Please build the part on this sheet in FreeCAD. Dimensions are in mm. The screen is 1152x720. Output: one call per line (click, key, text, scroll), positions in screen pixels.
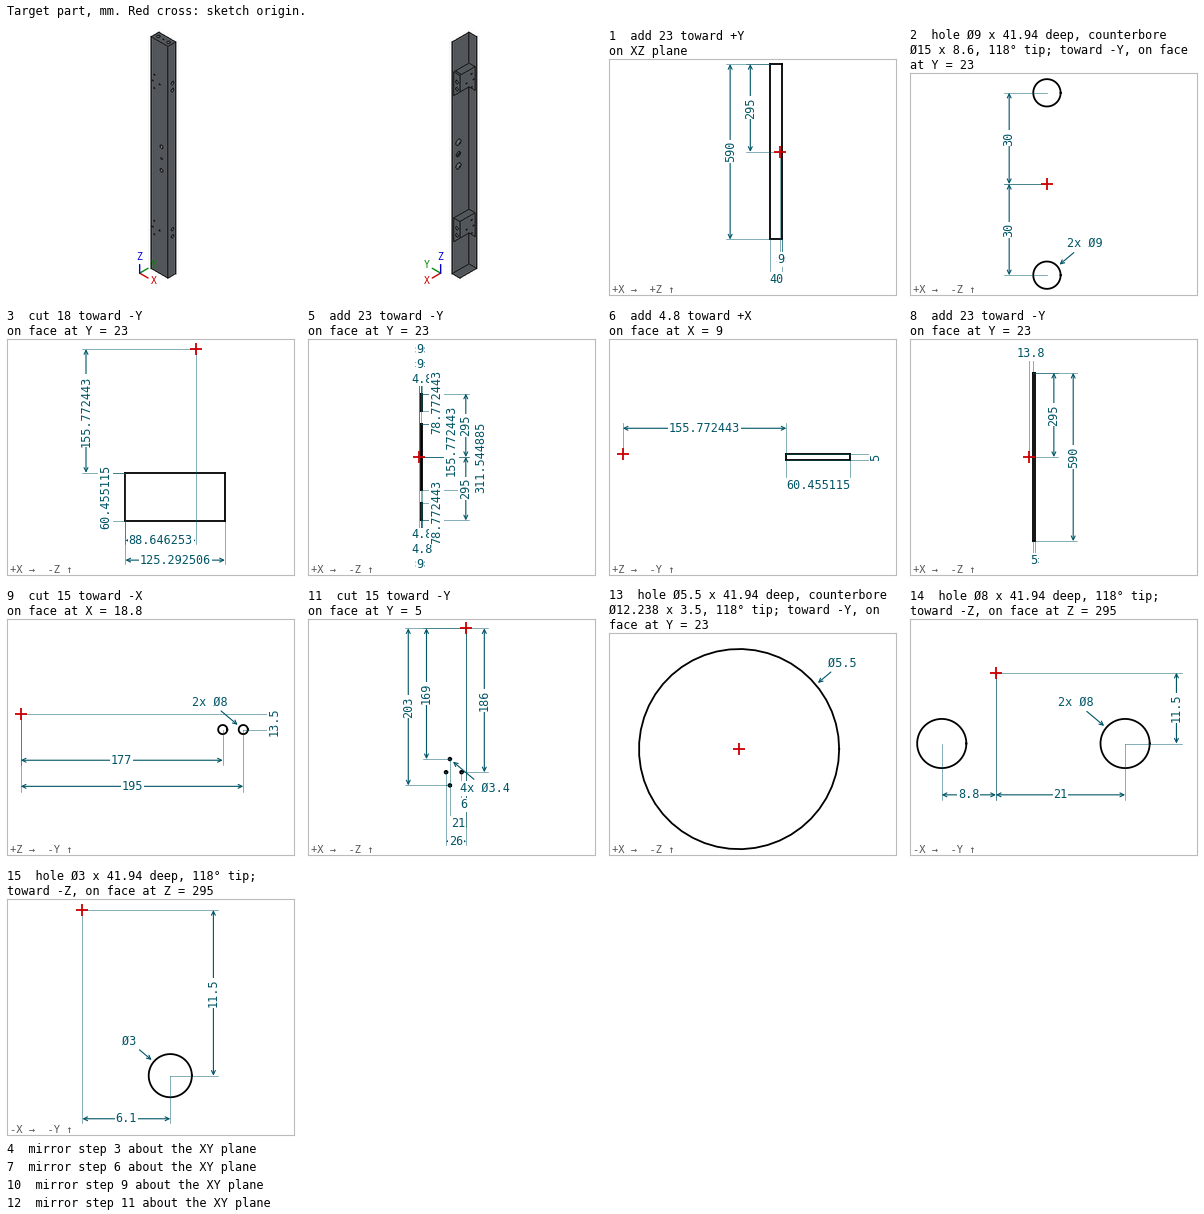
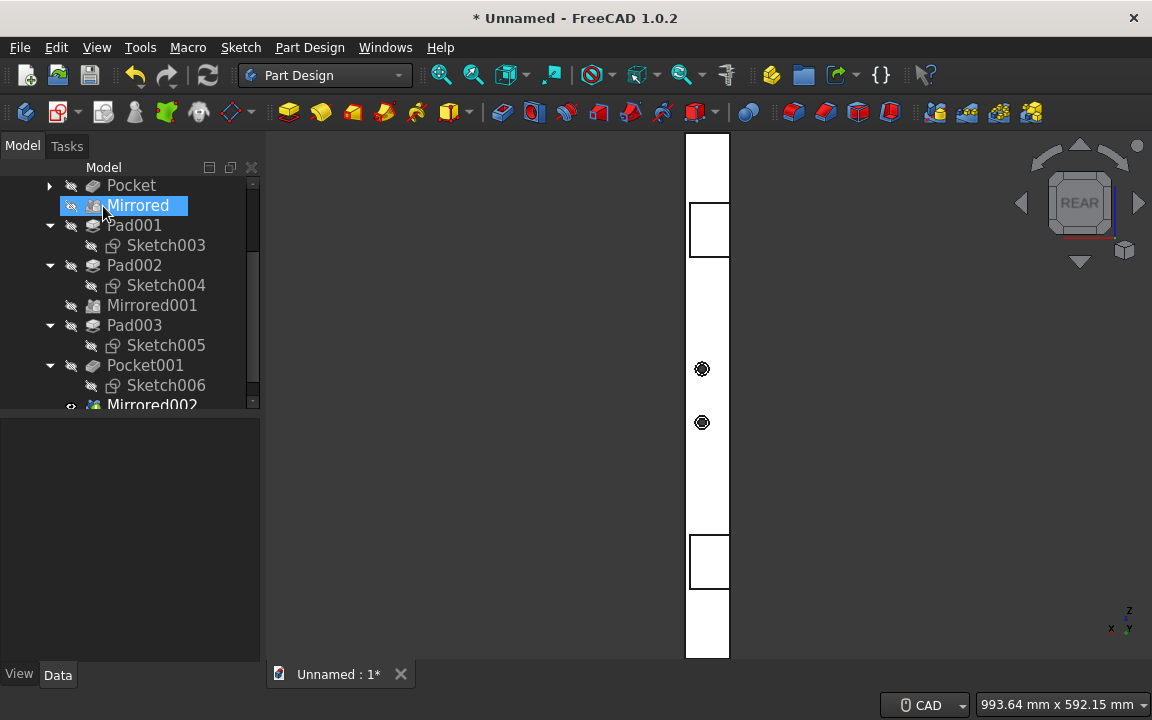
click(710, 229)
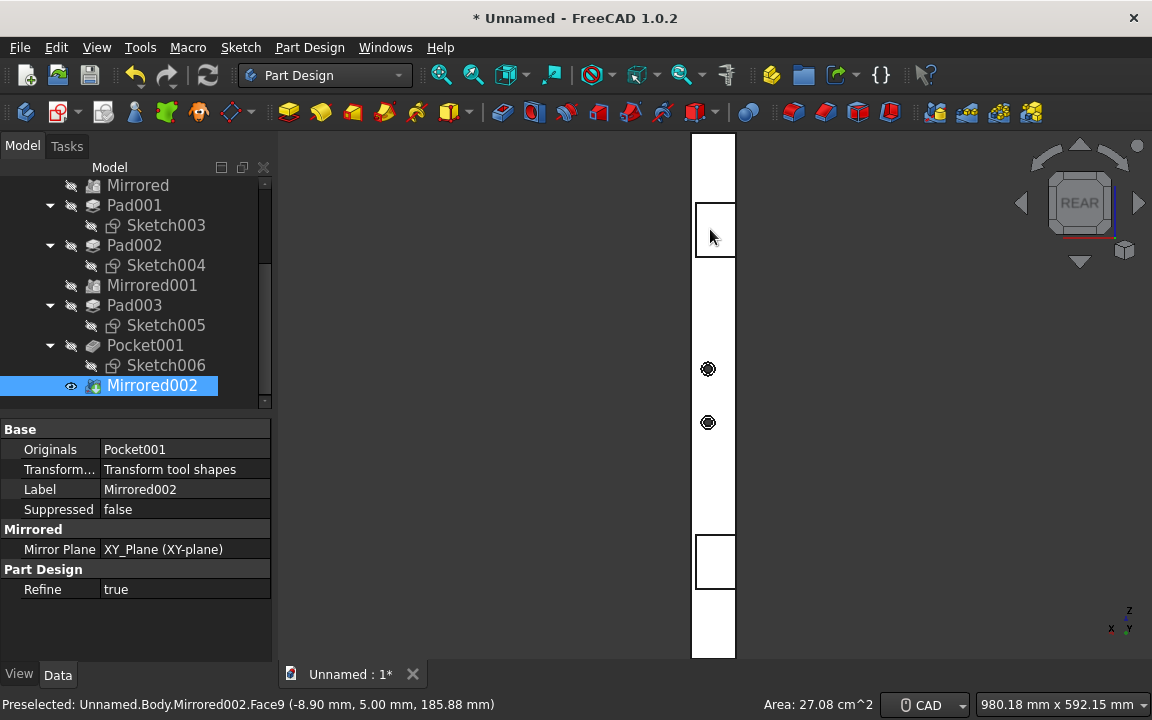
click(58, 112)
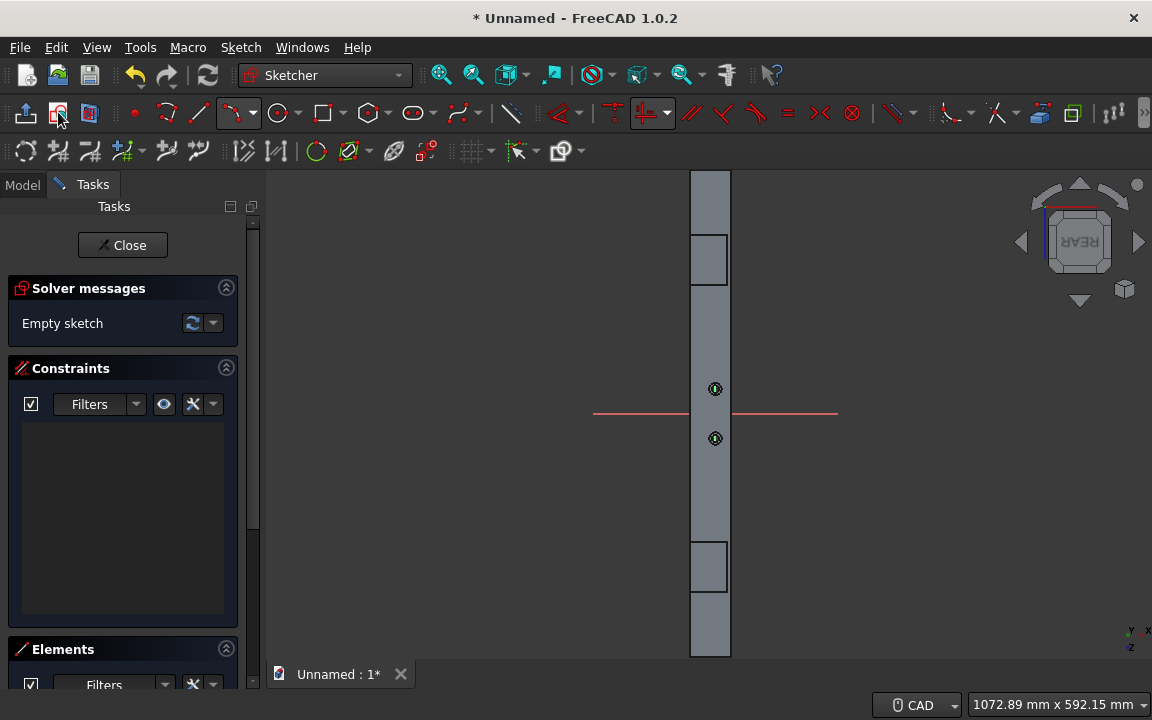
scroll(710, 586, up, 11)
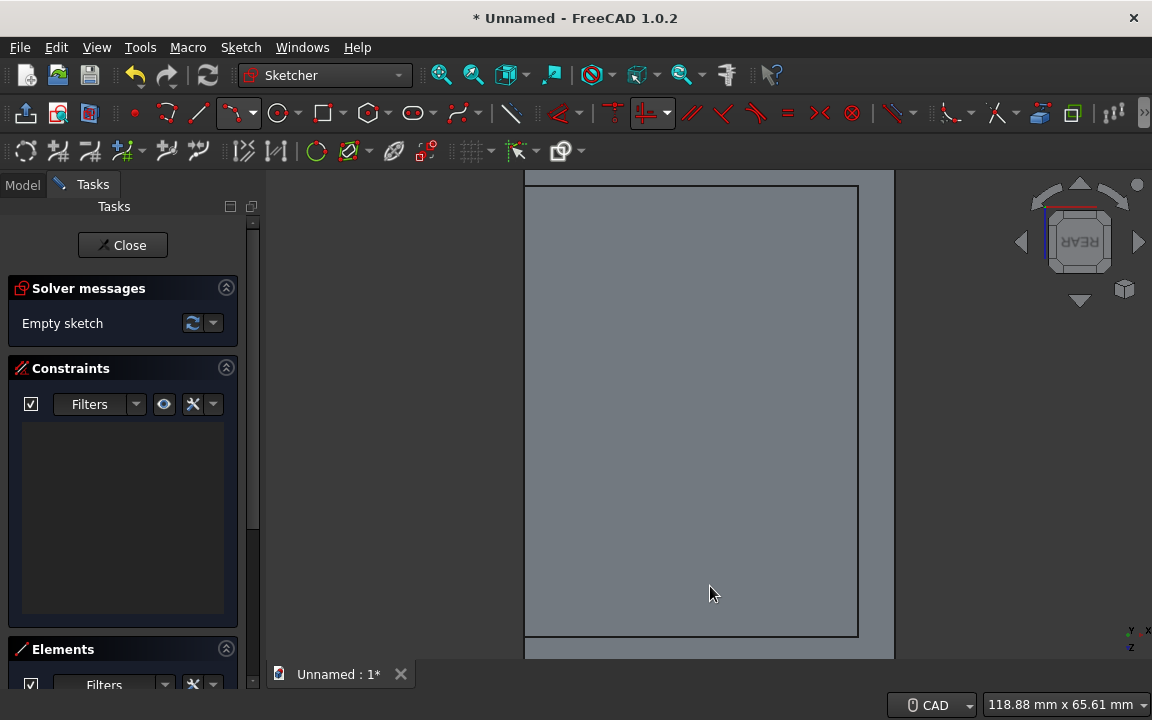
click(278, 114)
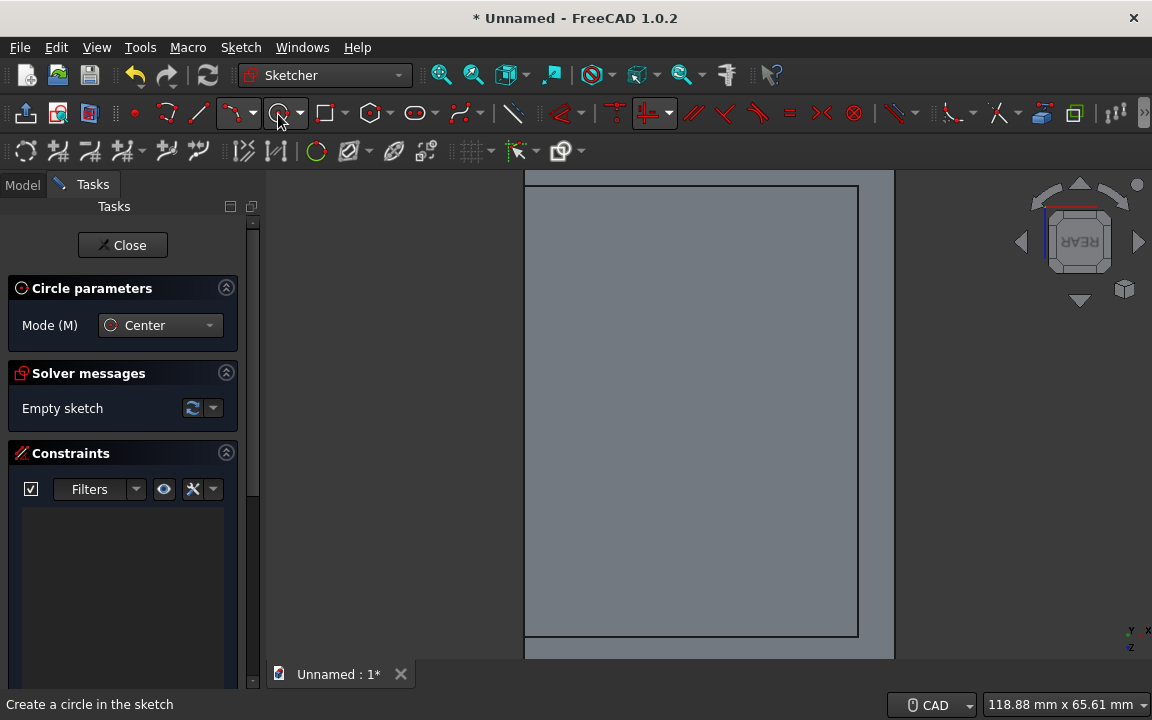
scroll(598, 285, up, 3)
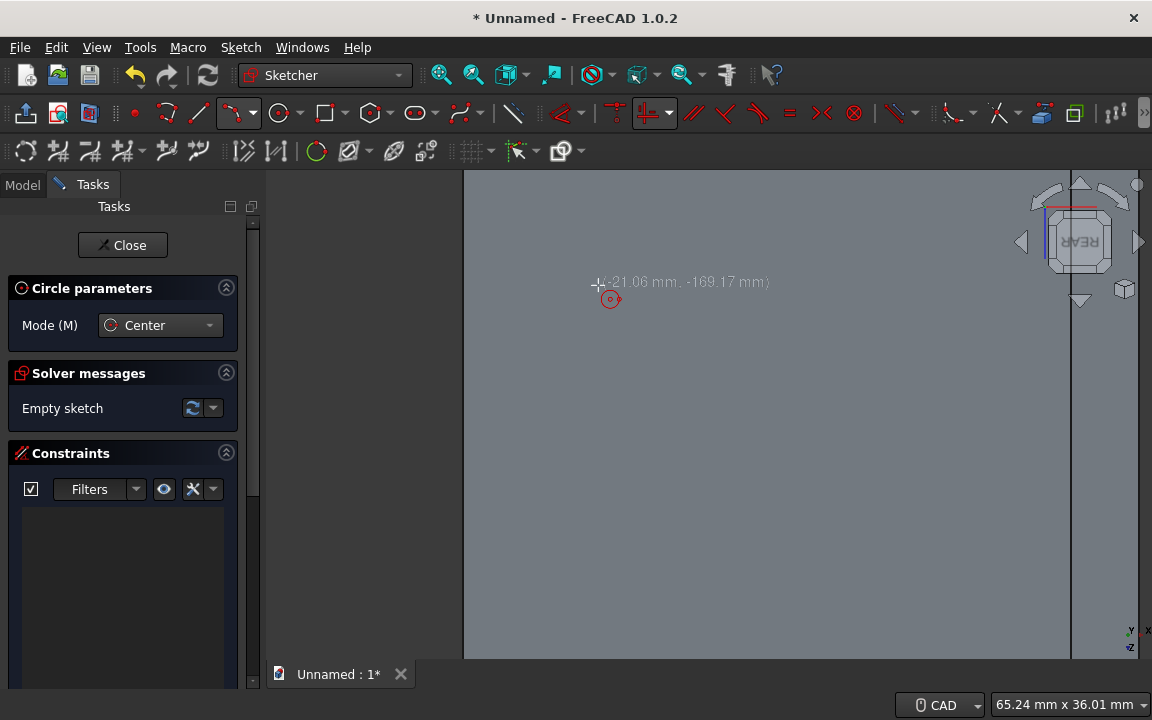
click(598, 284)
click(615, 268)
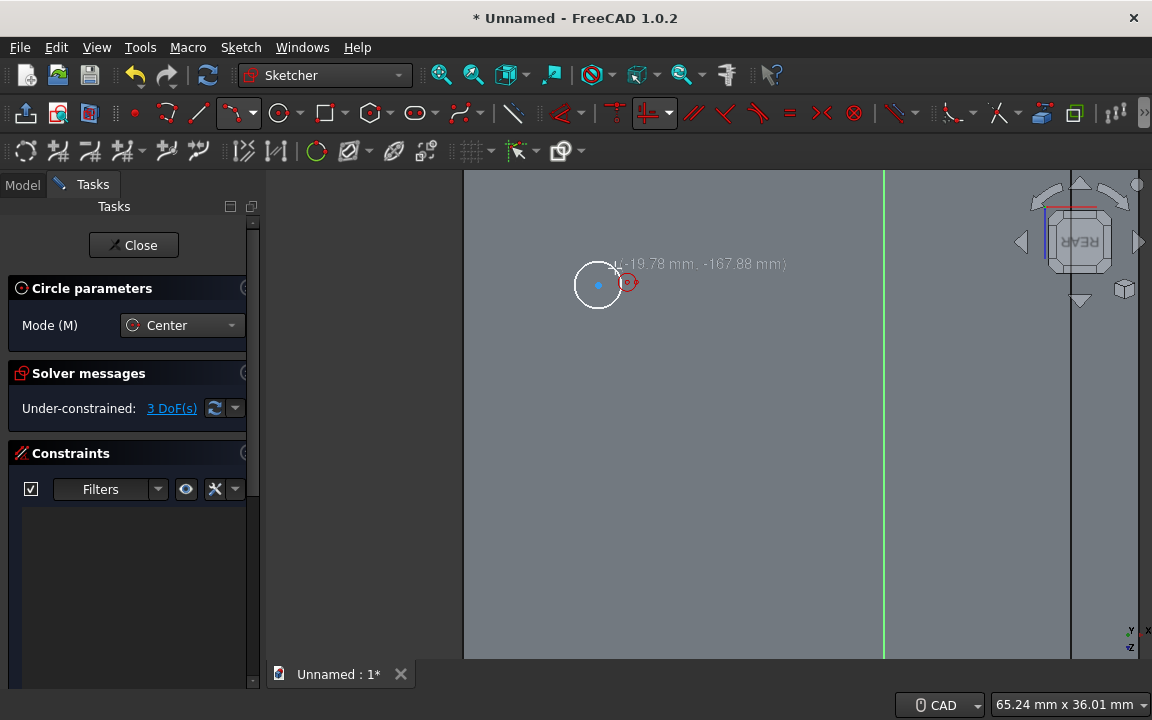
click(802, 515)
click(818, 499)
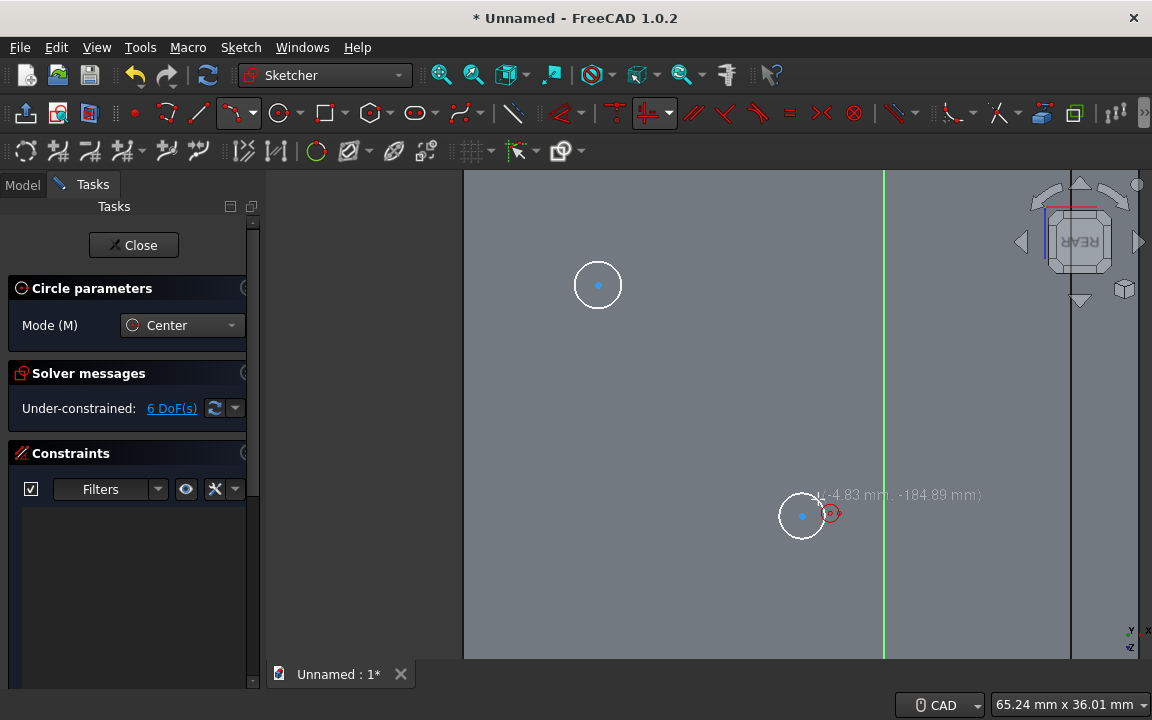
click(531, 515)
click(547, 499)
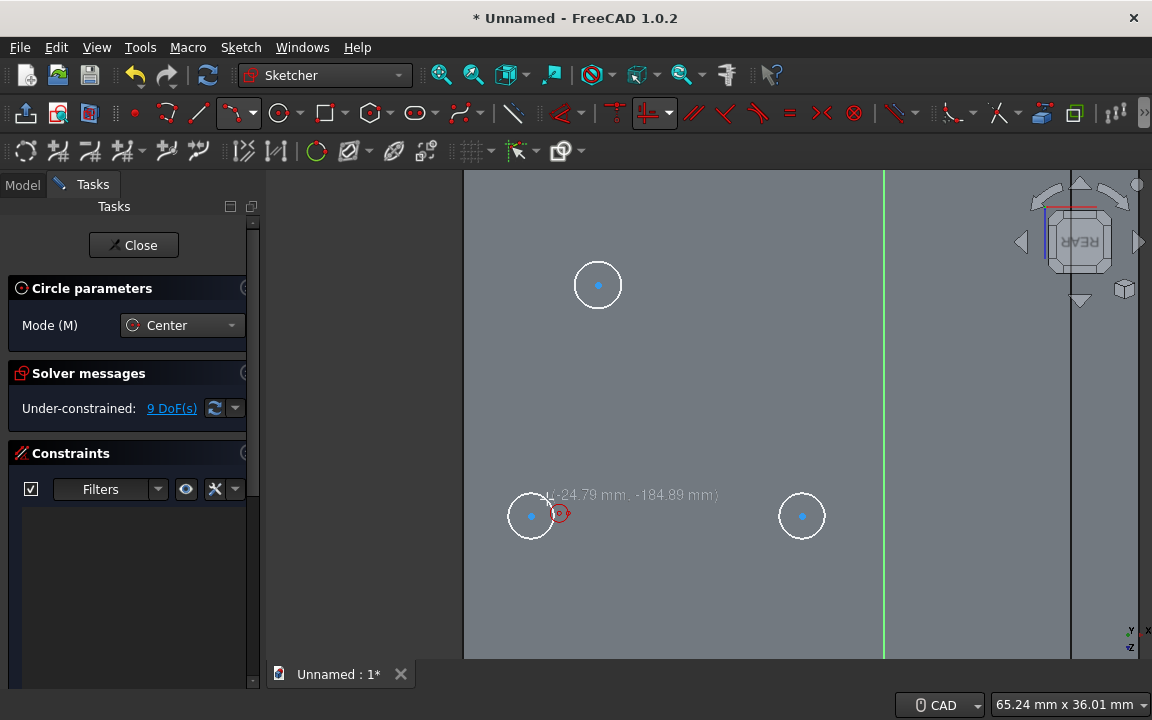
scroll(609, 292, down, 3)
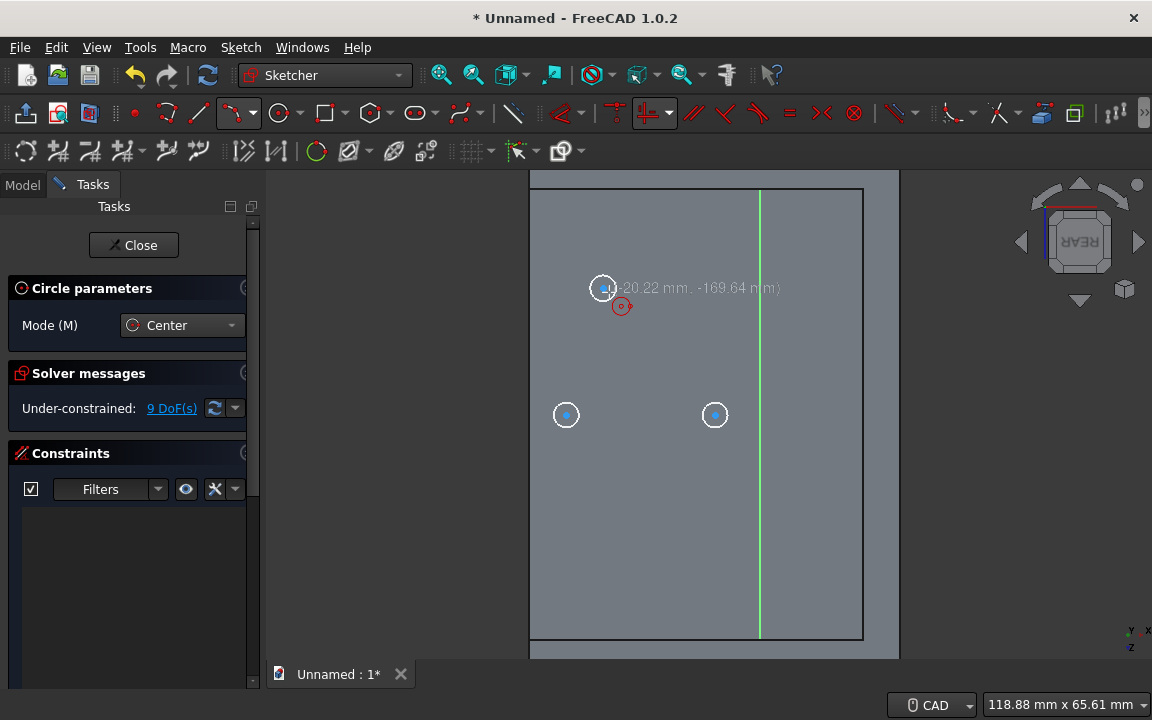
scroll(603, 541, up, 3)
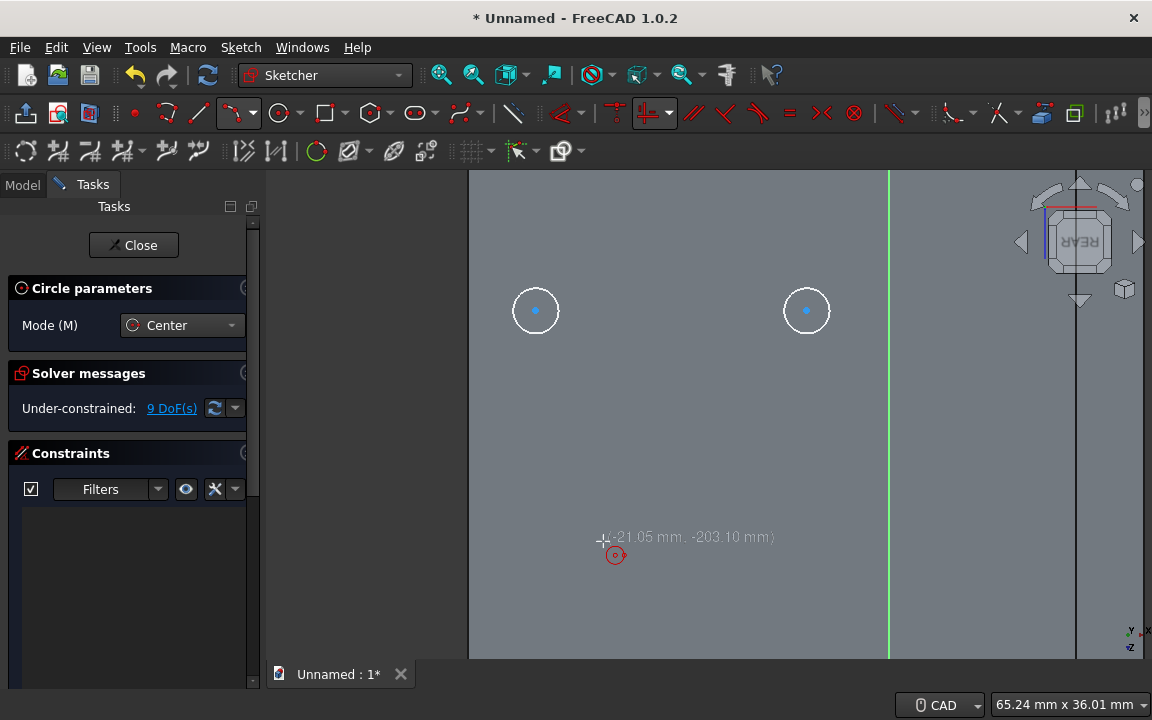
click(603, 541)
click(620, 525)
key(Escape)